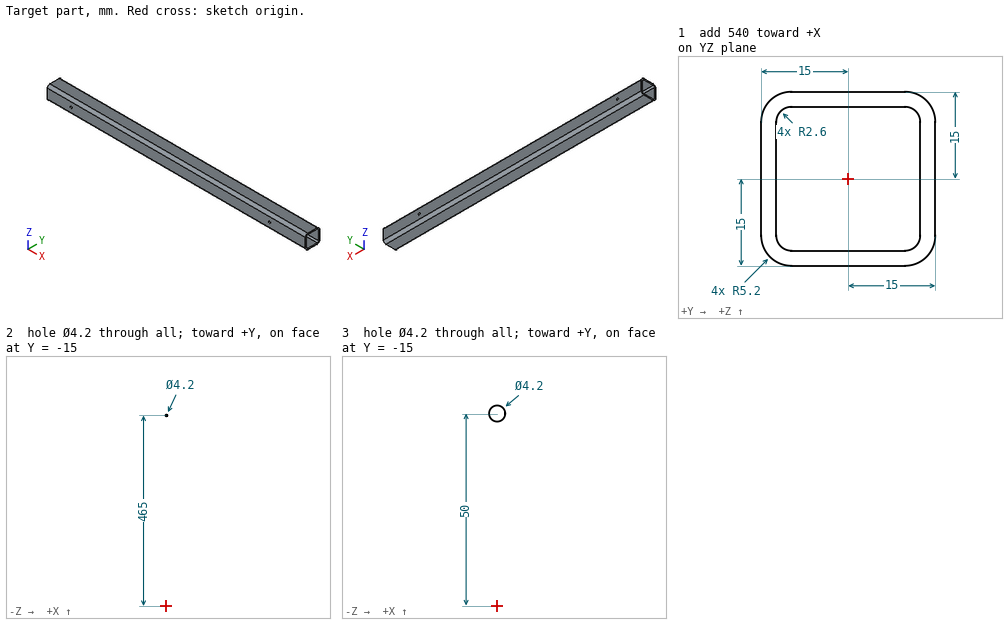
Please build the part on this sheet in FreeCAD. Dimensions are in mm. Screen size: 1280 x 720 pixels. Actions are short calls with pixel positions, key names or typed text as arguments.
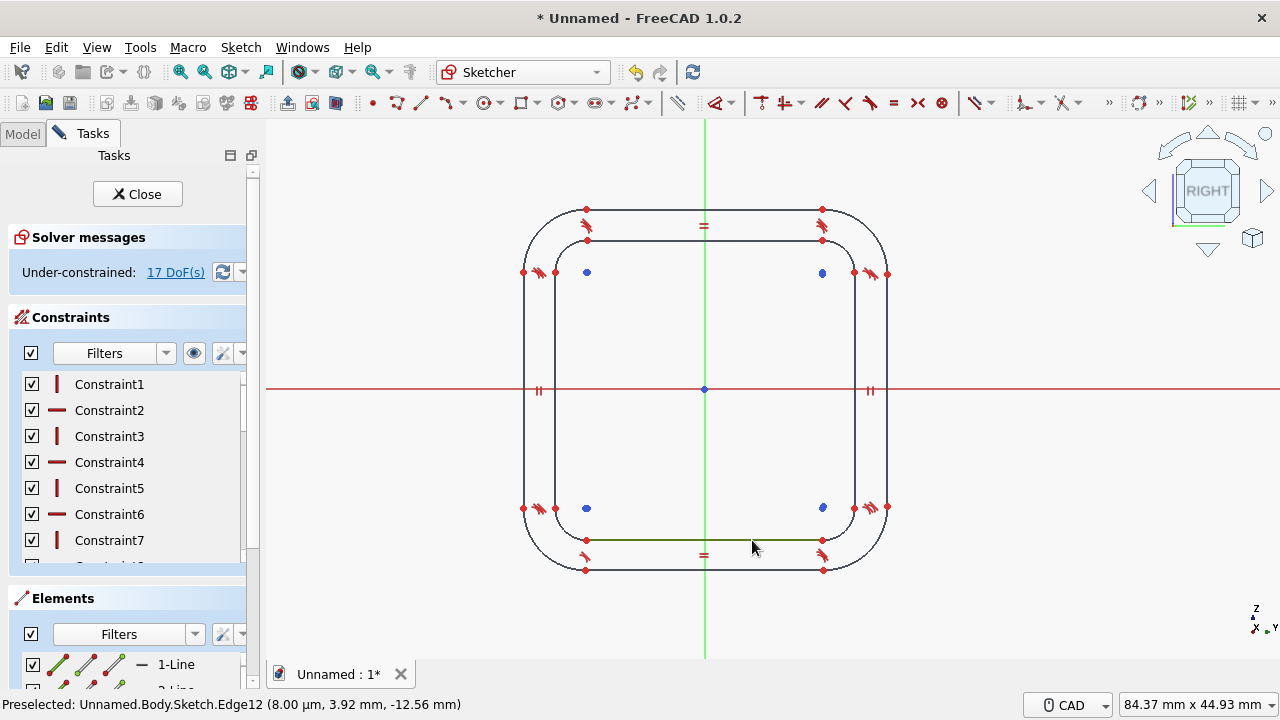
click(559, 523)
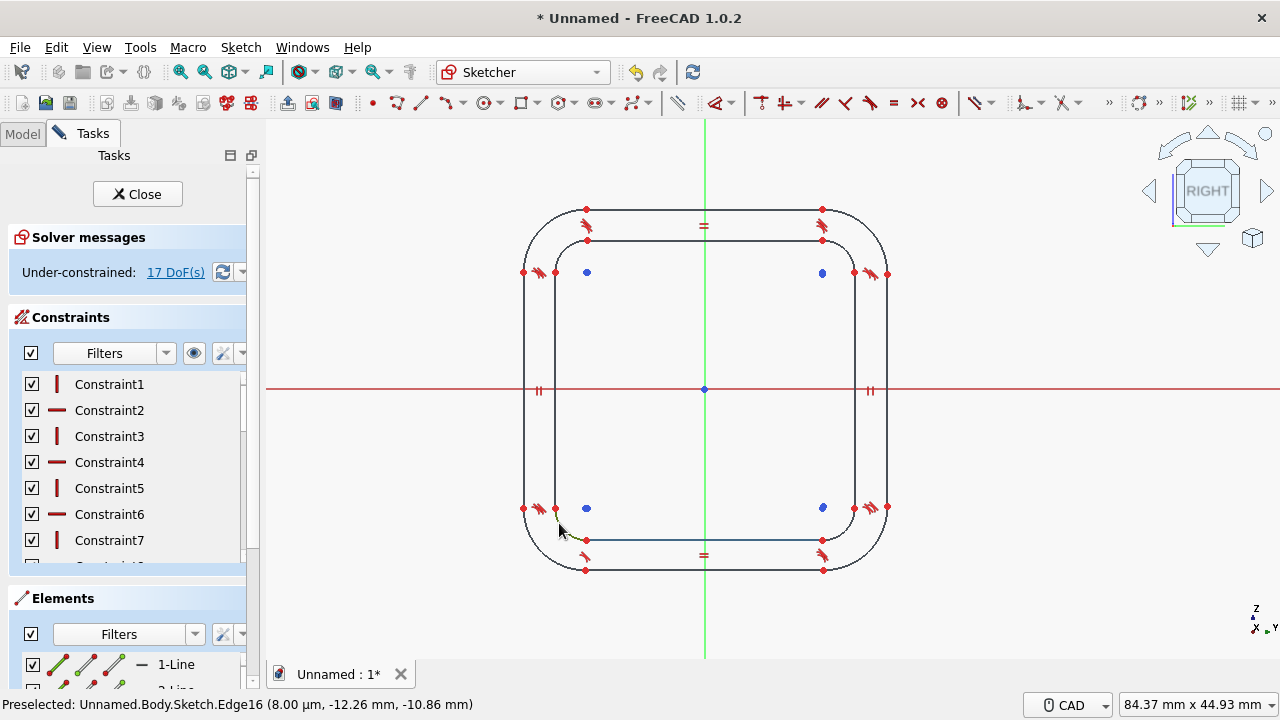
key(t)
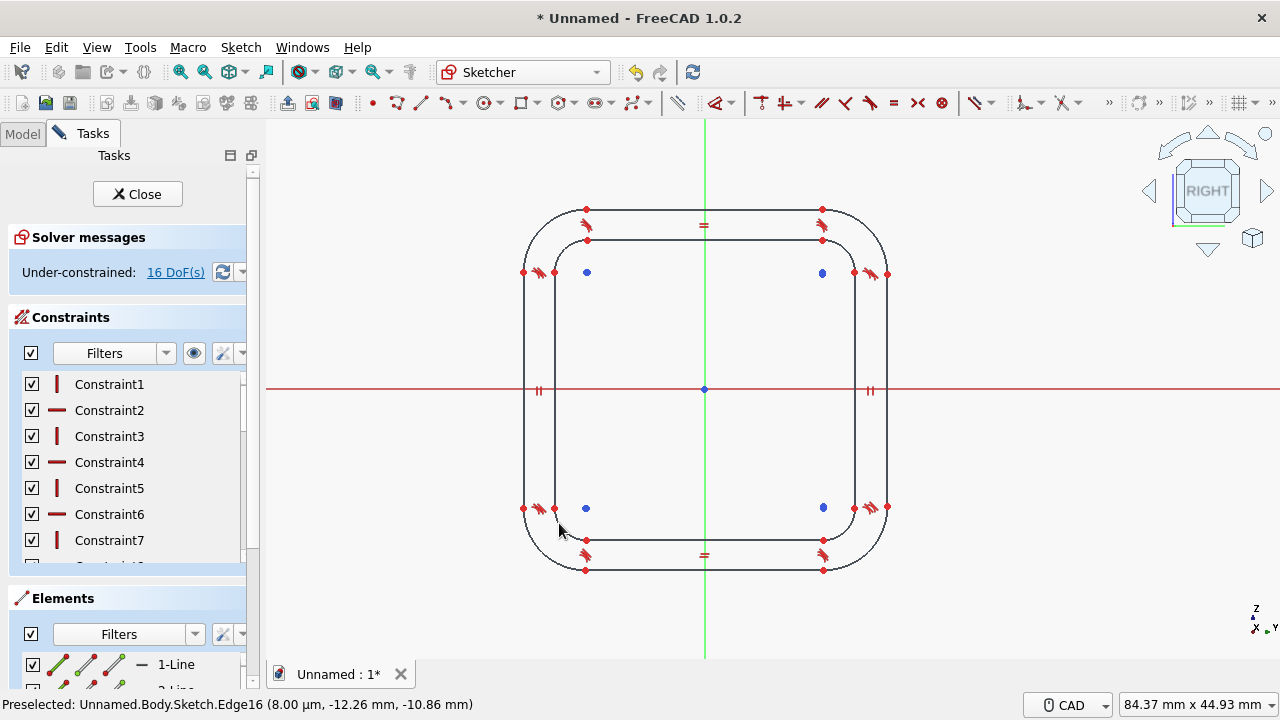
click(558, 216)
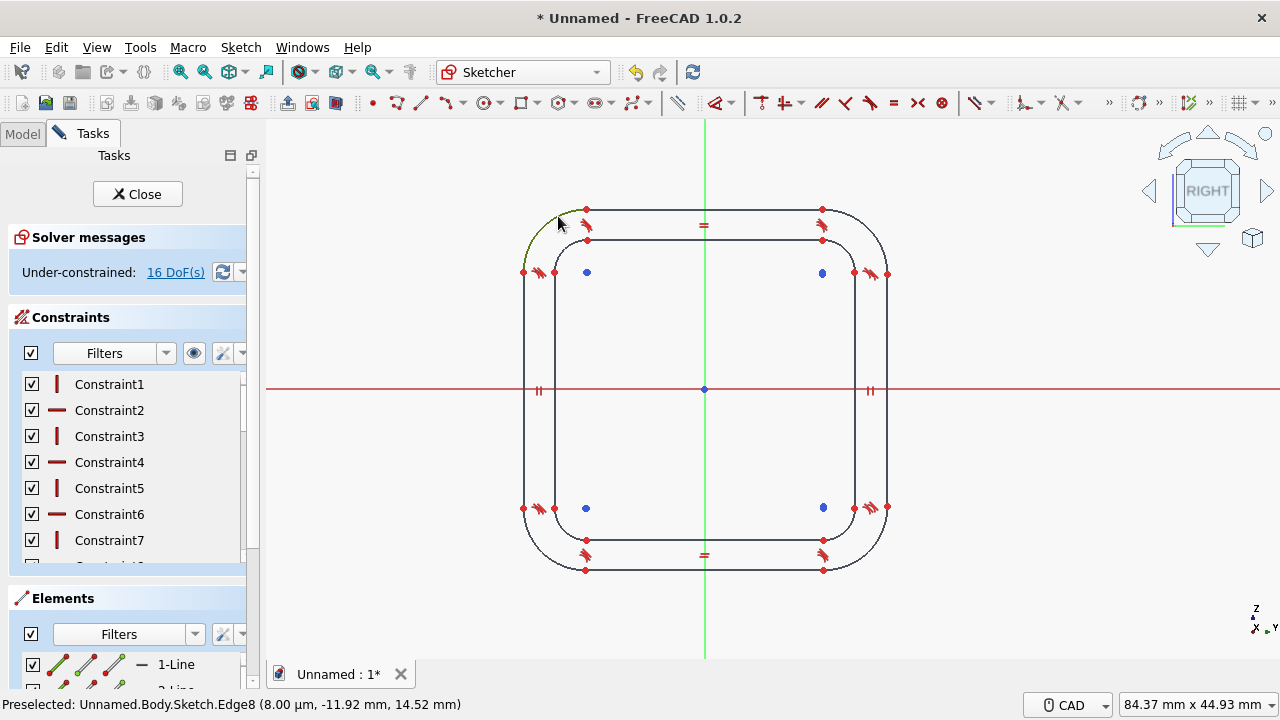
click(572, 244)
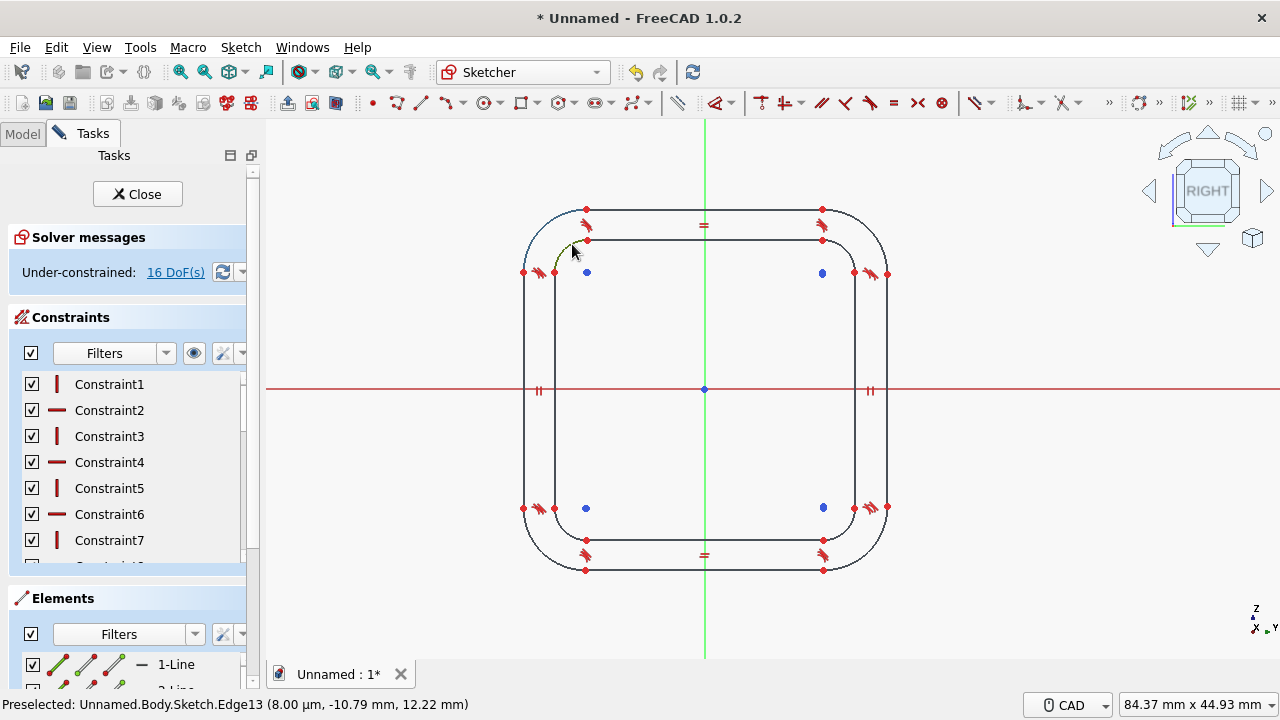
click(762, 104)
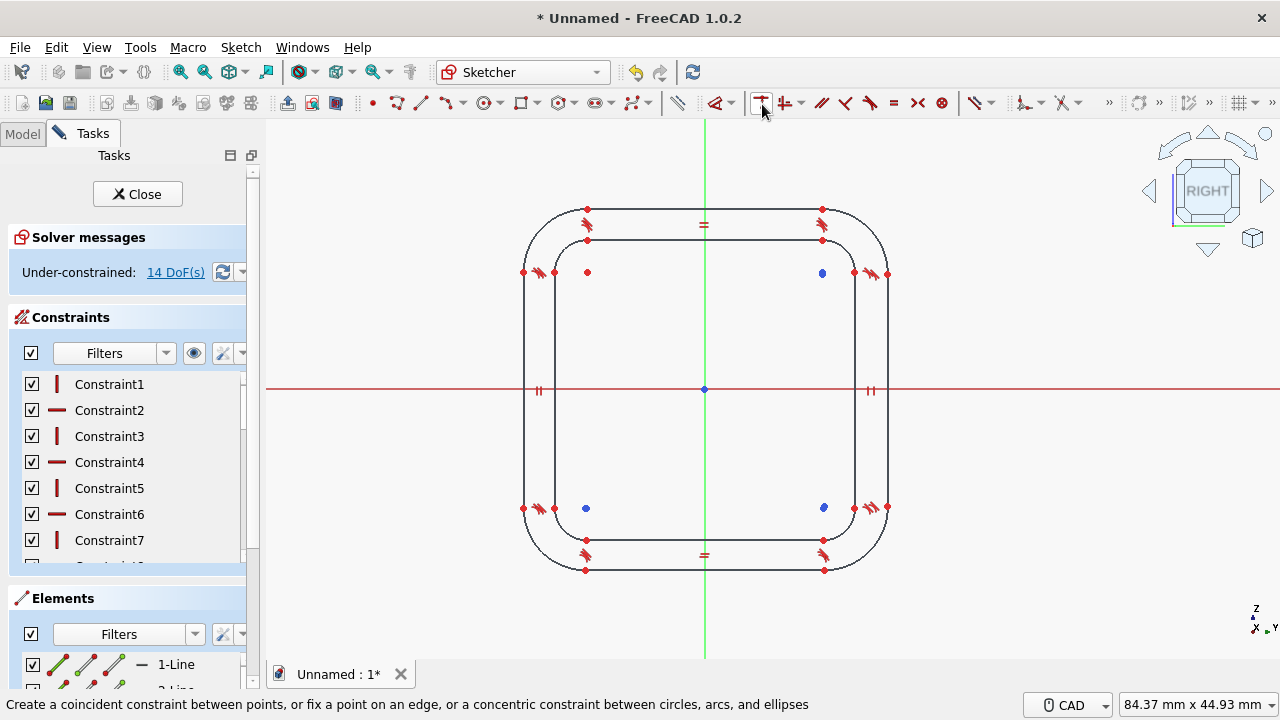
click(881, 245)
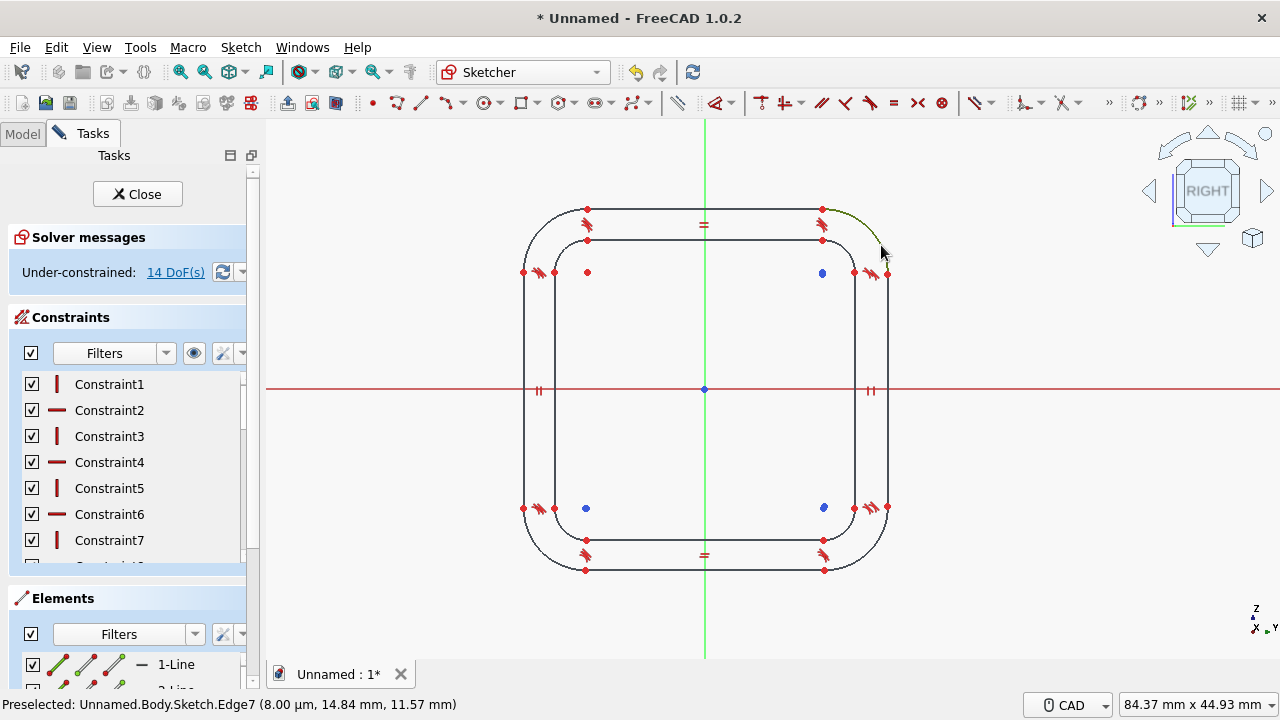
click(851, 258)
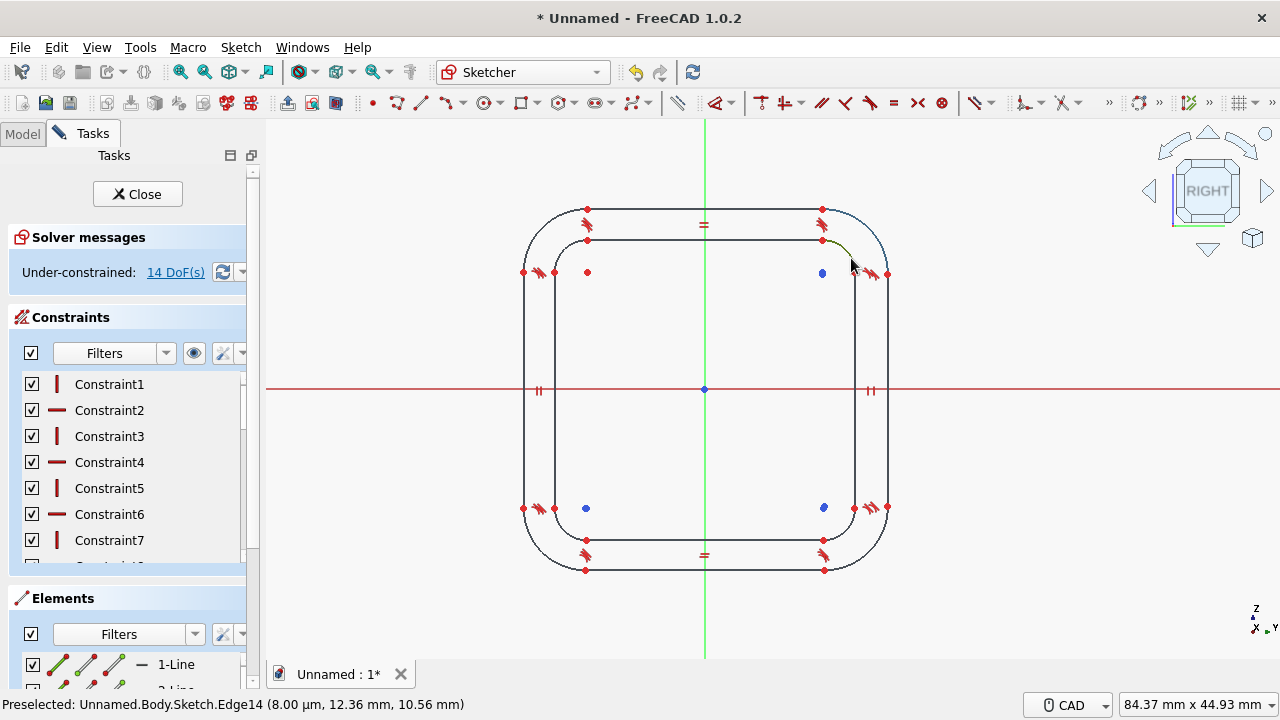
click(762, 104)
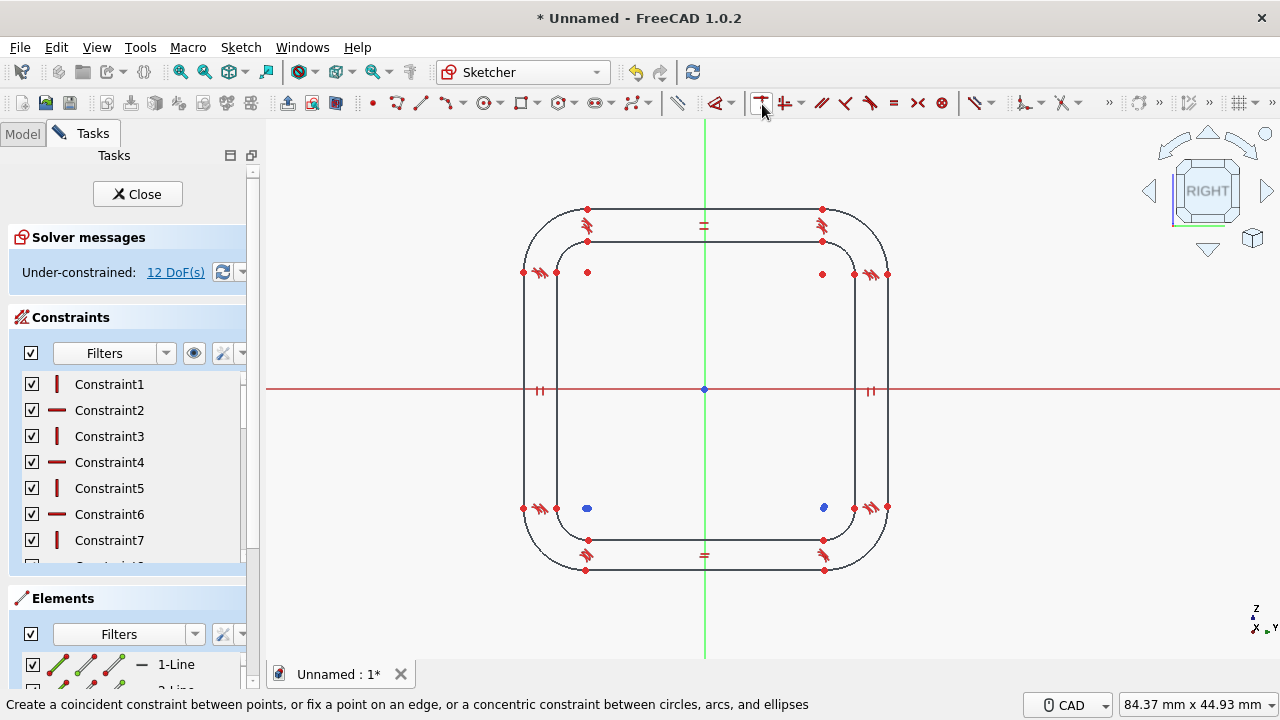
click(853, 563)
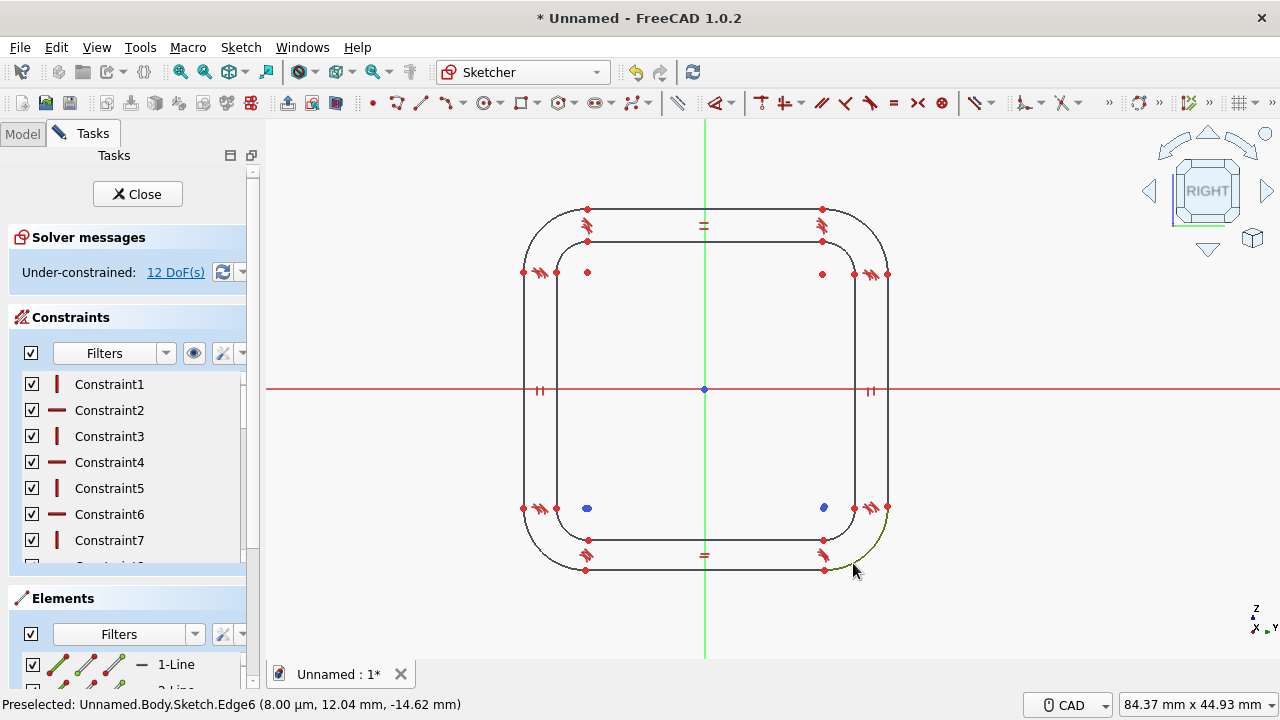
click(838, 537)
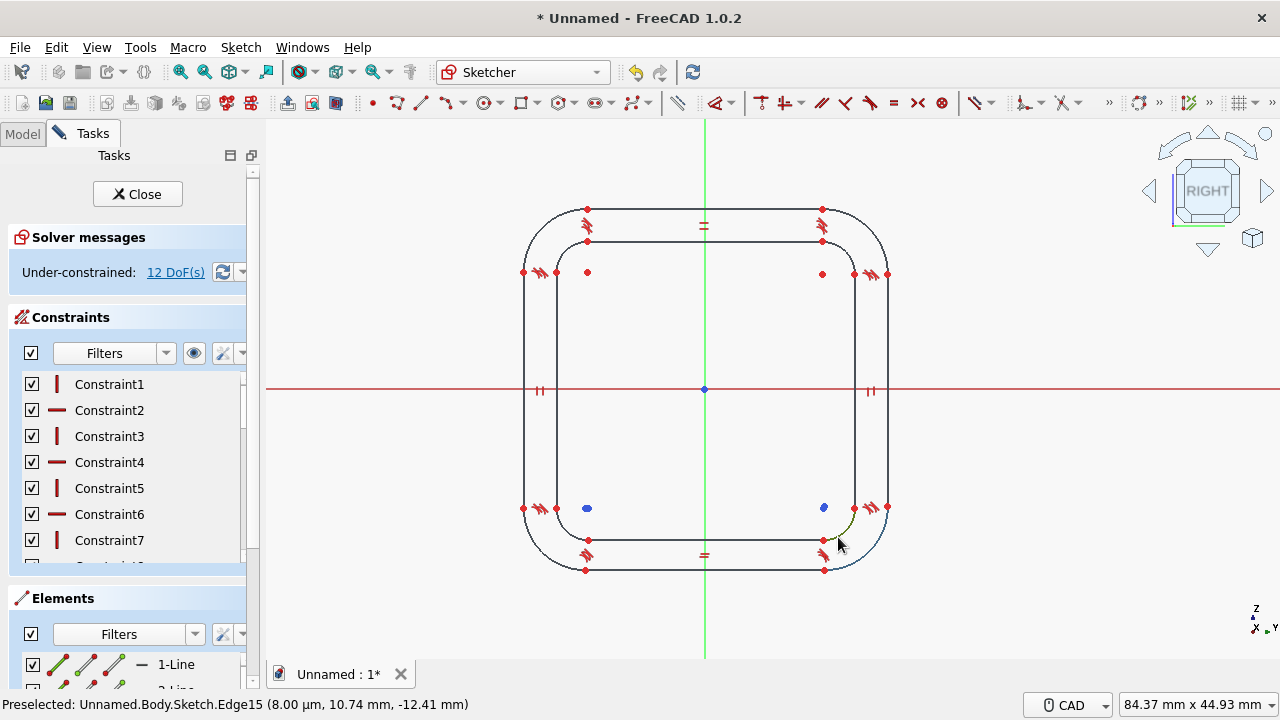
click(762, 104)